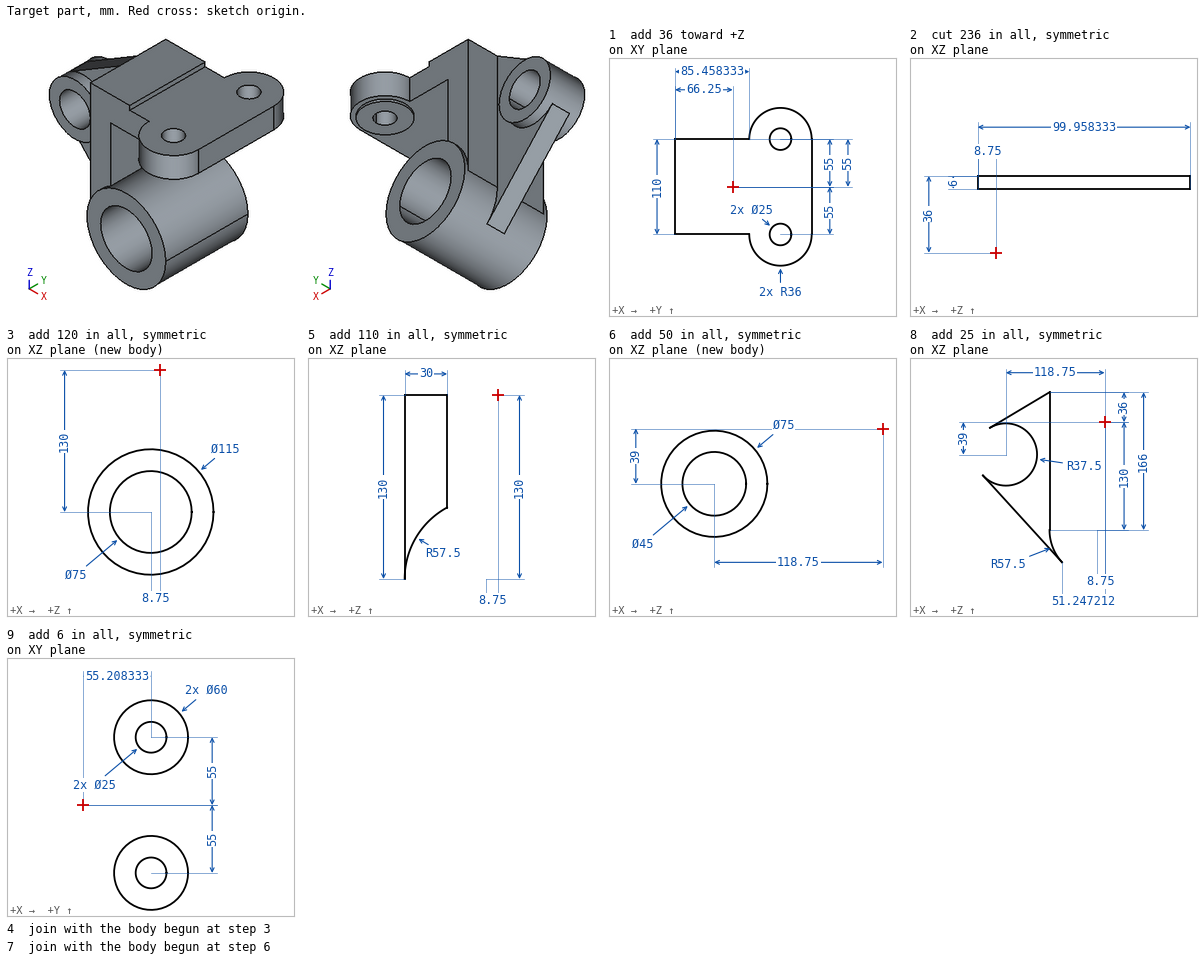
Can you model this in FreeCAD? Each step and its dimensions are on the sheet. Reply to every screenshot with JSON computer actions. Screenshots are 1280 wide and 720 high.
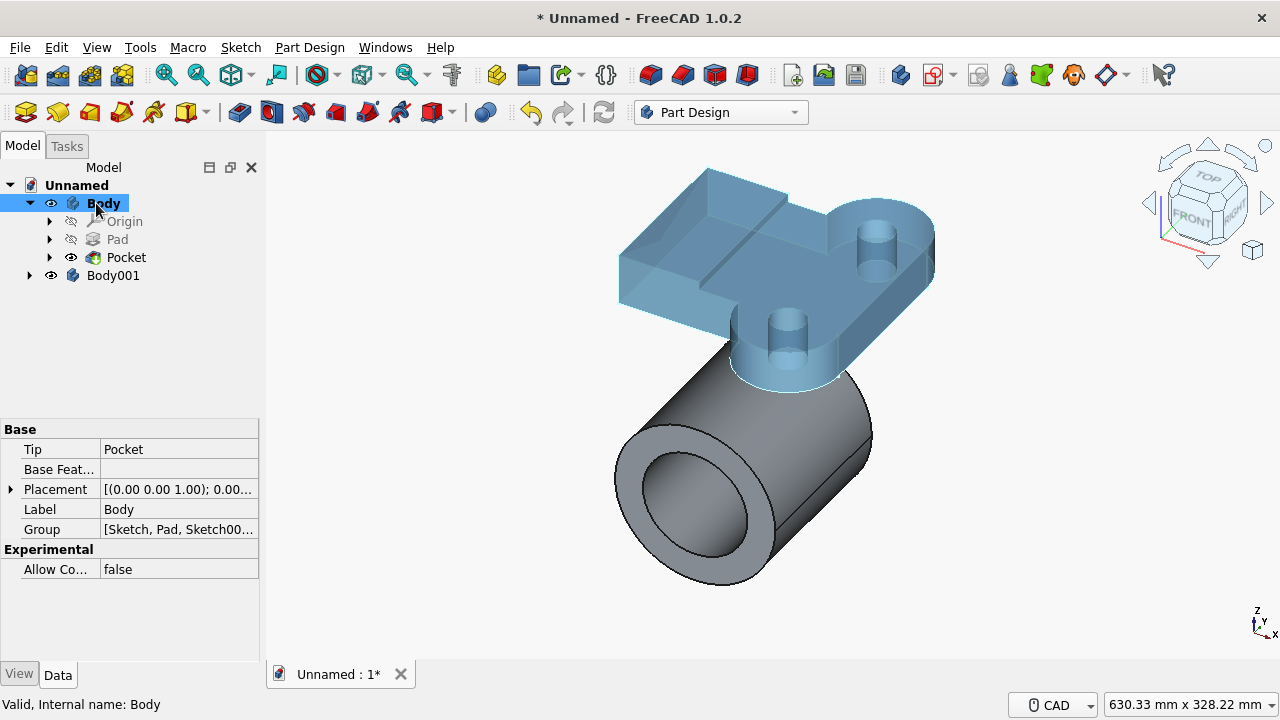
{"action": "left_click", "coordinate": [96, 203]}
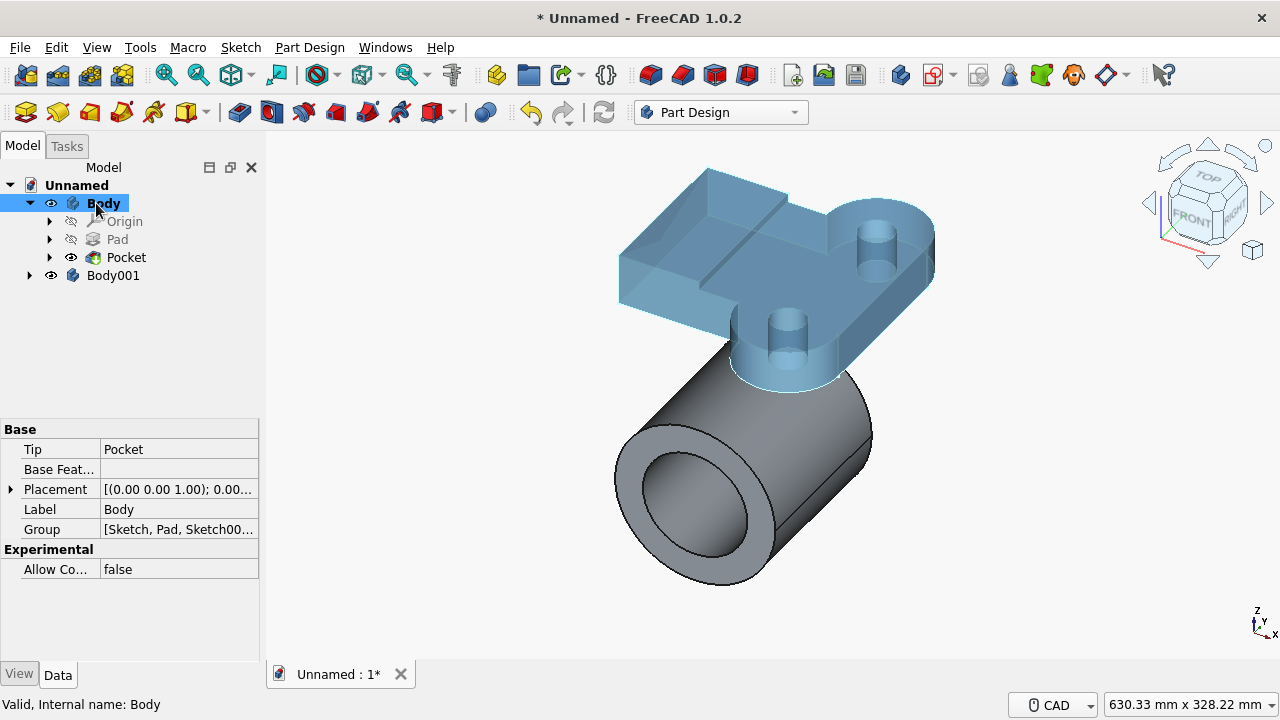
{"action": "left_click", "coordinate": [146, 569]}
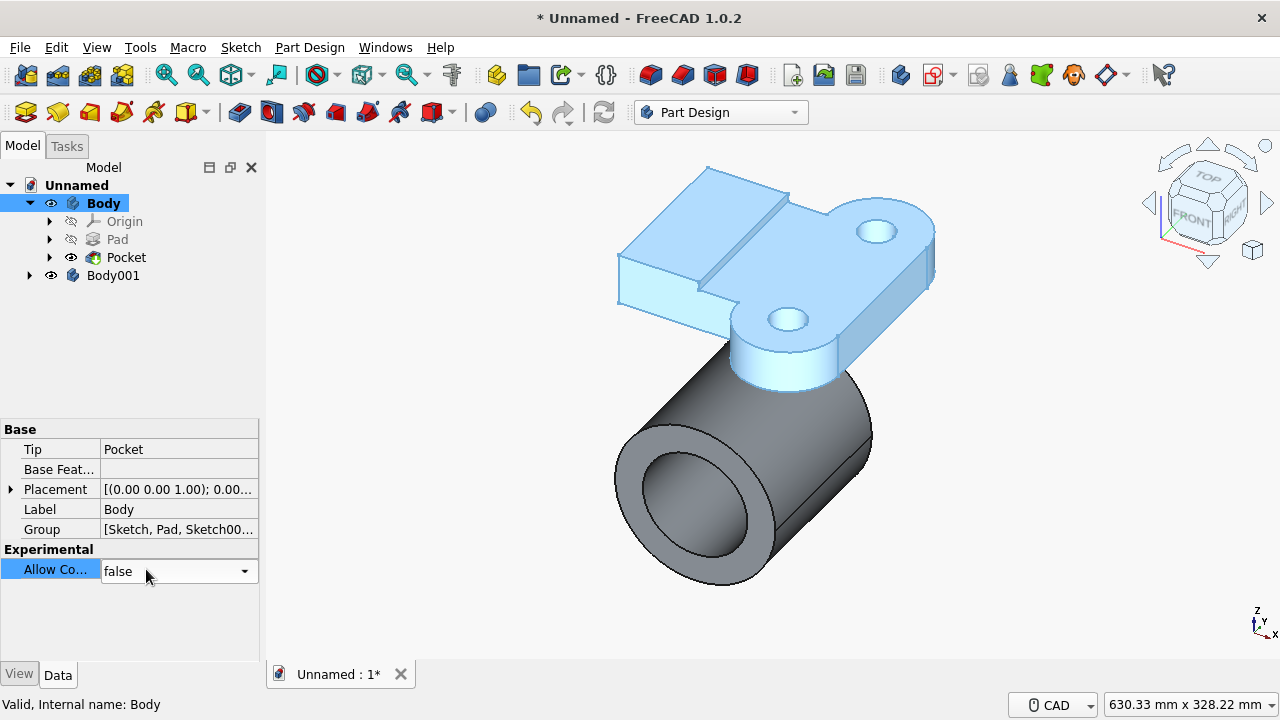
{"action": "left_click", "coordinate": [146, 569]}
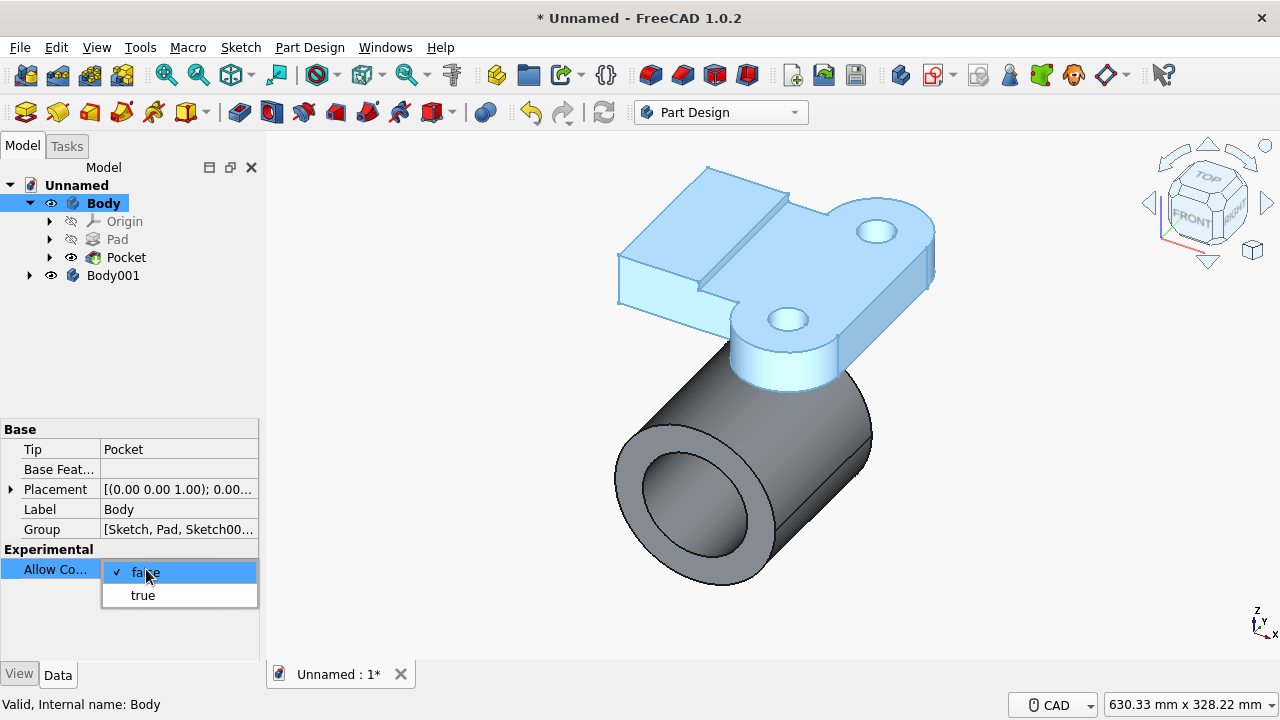
{"action": "left_click", "coordinate": [179, 596]}
{"action": "key", "text": "Return"}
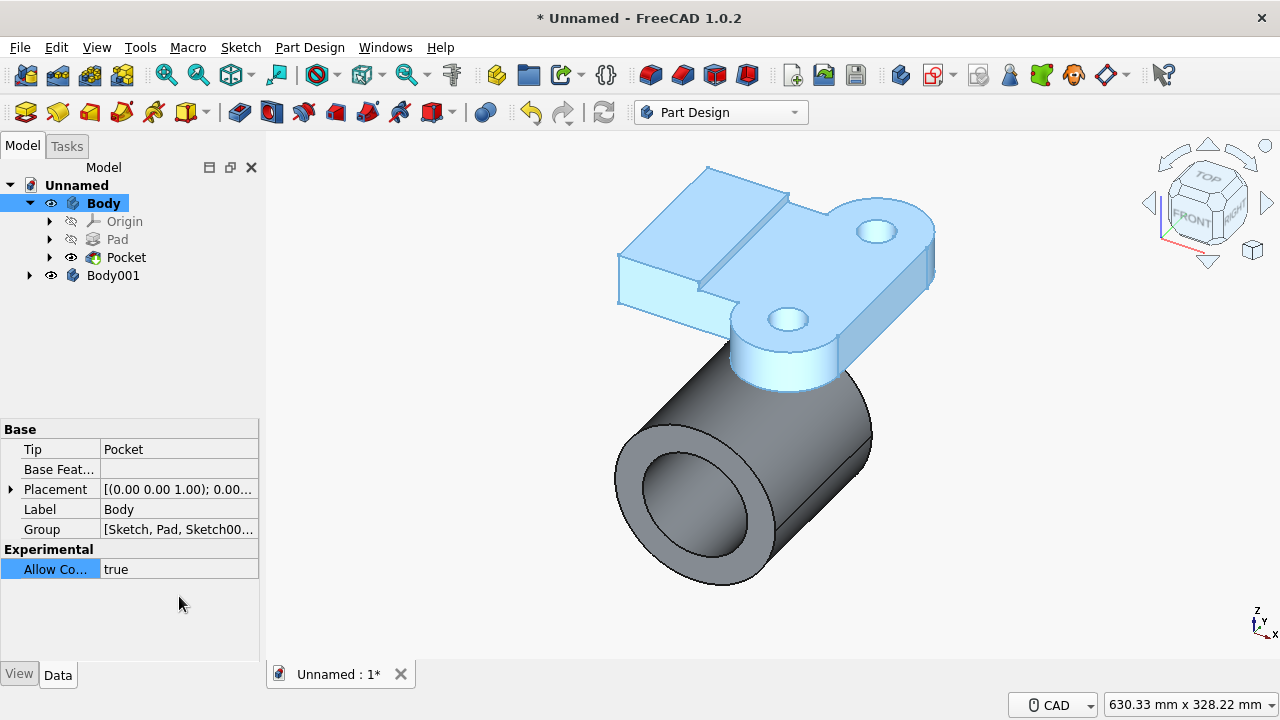
{"action": "left_click", "coordinate": [96, 275]}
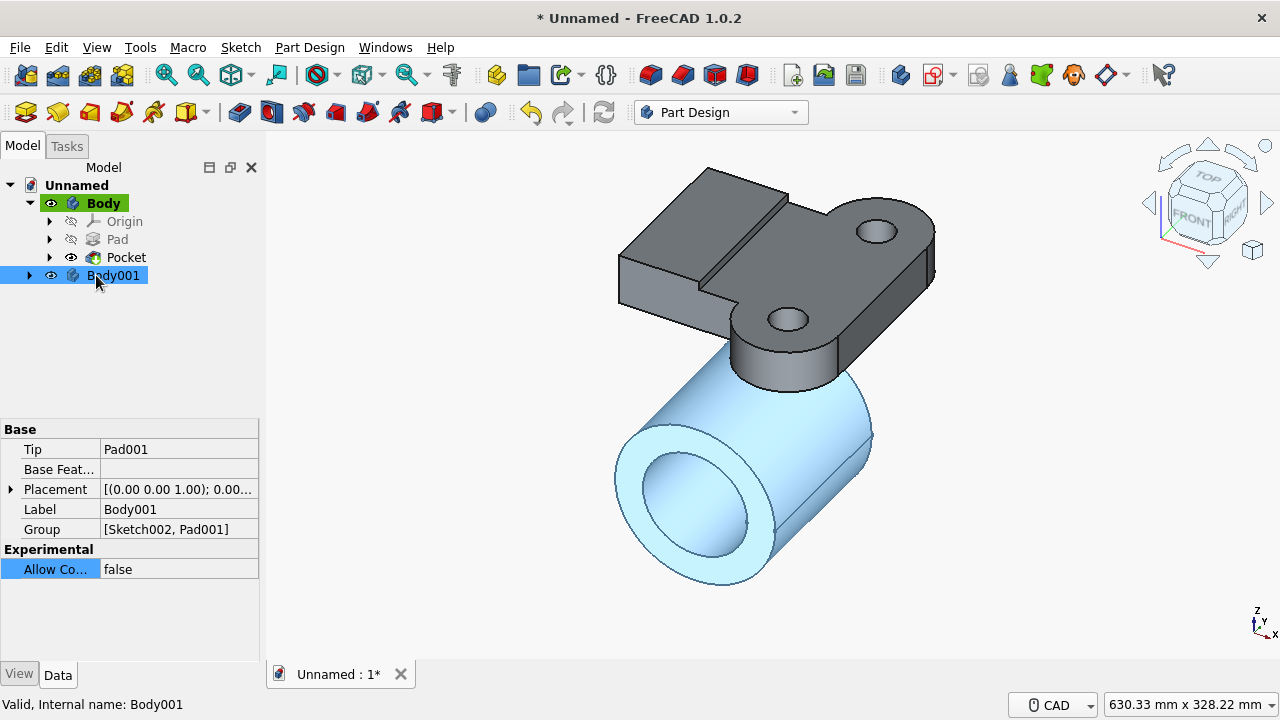
{"action": "left_click", "coordinate": [486, 112]}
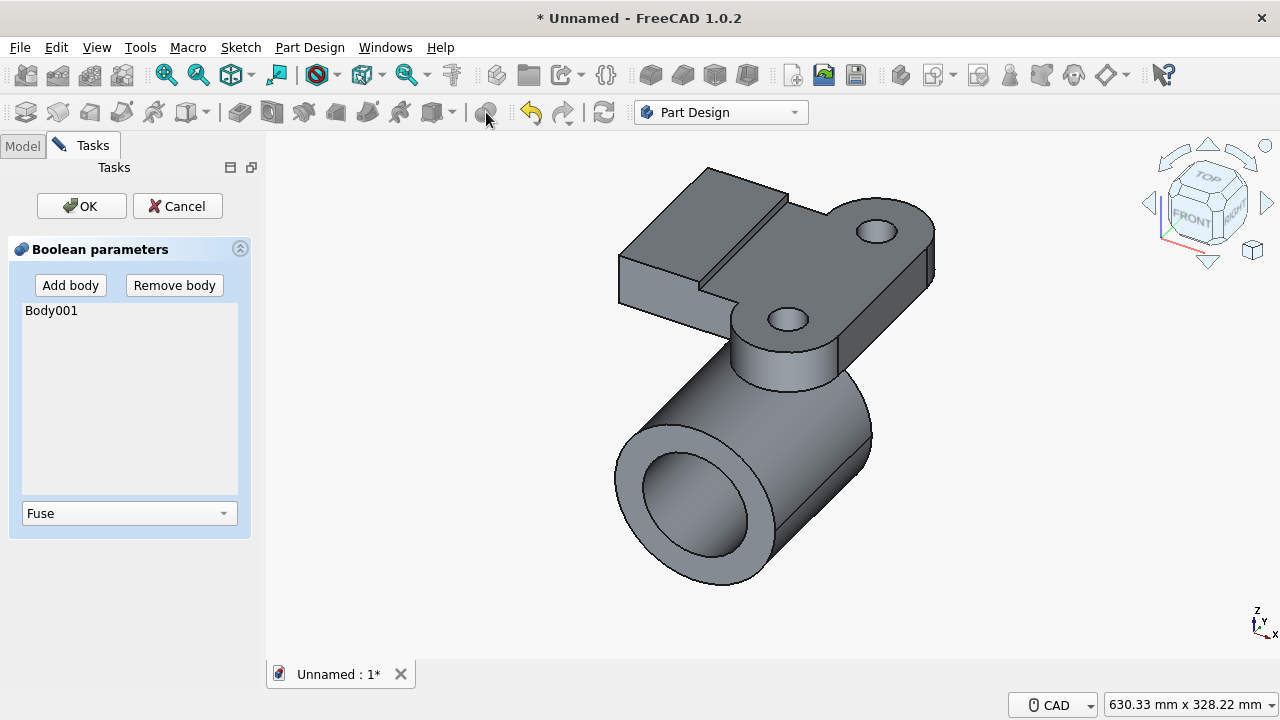
{"action": "left_click", "coordinate": [82, 206]}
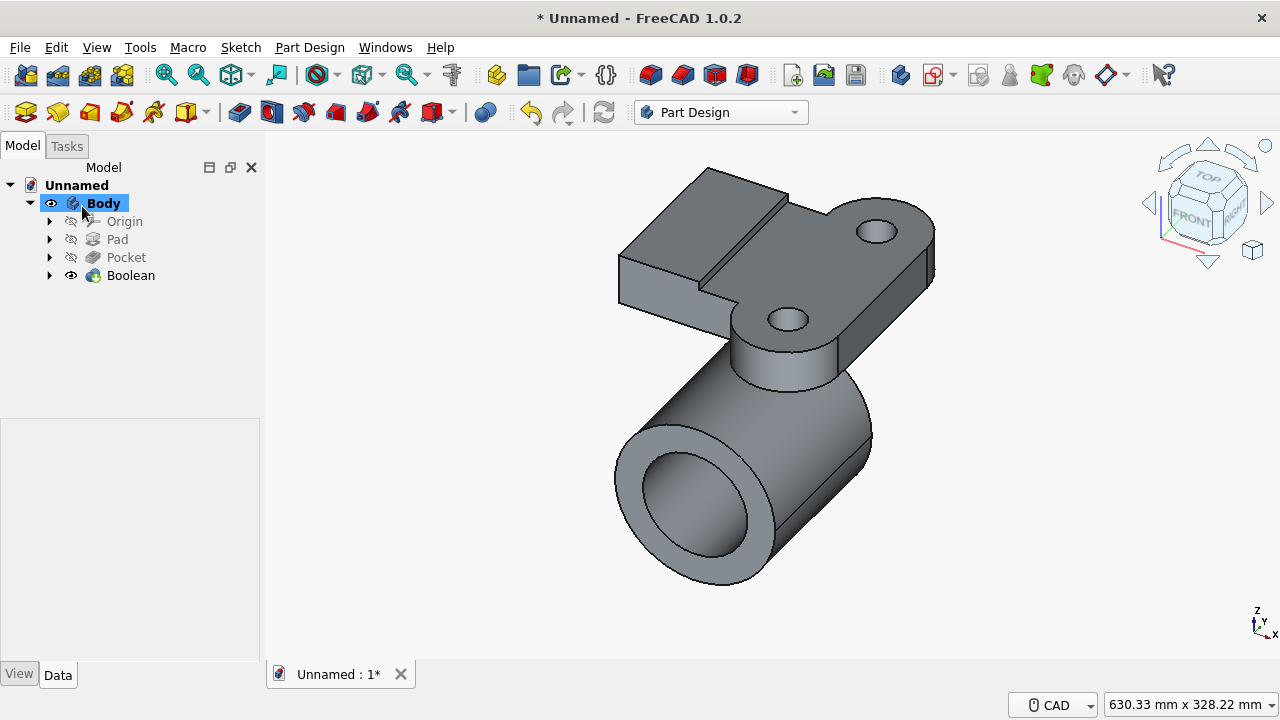
{"action": "left_click", "coordinate": [934, 76]}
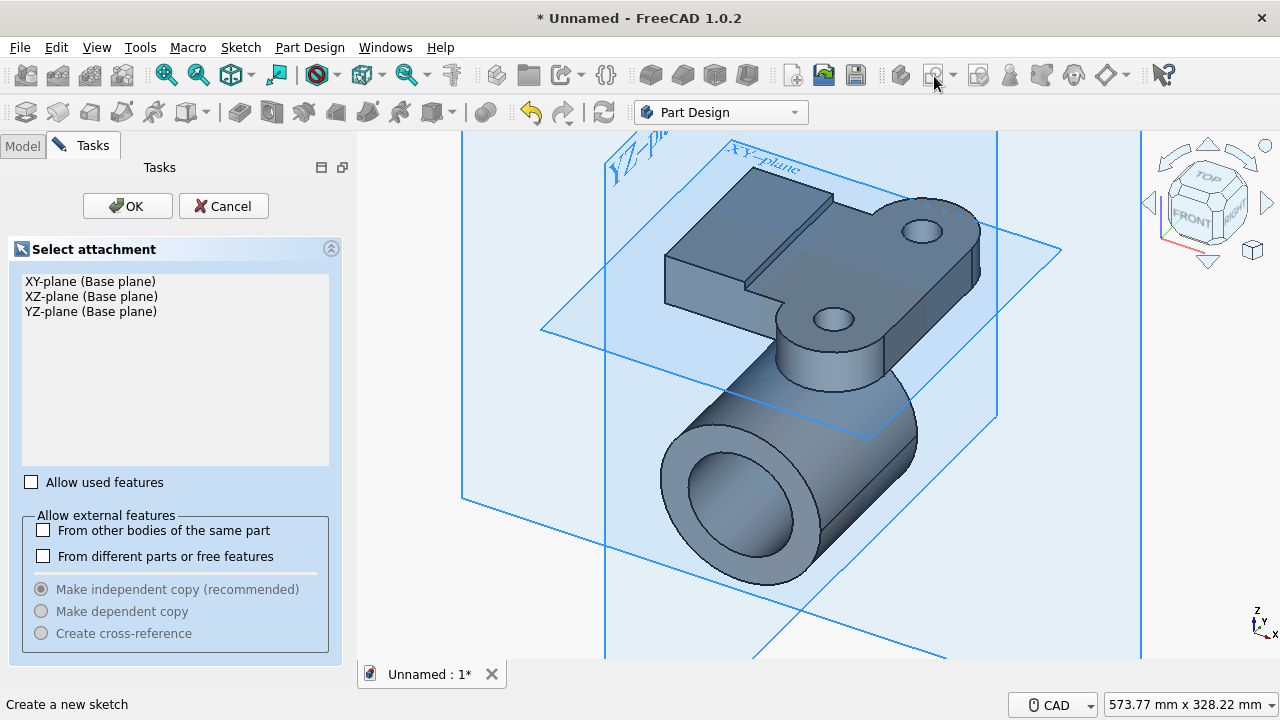
{"action": "left_click", "coordinate": [82, 296]}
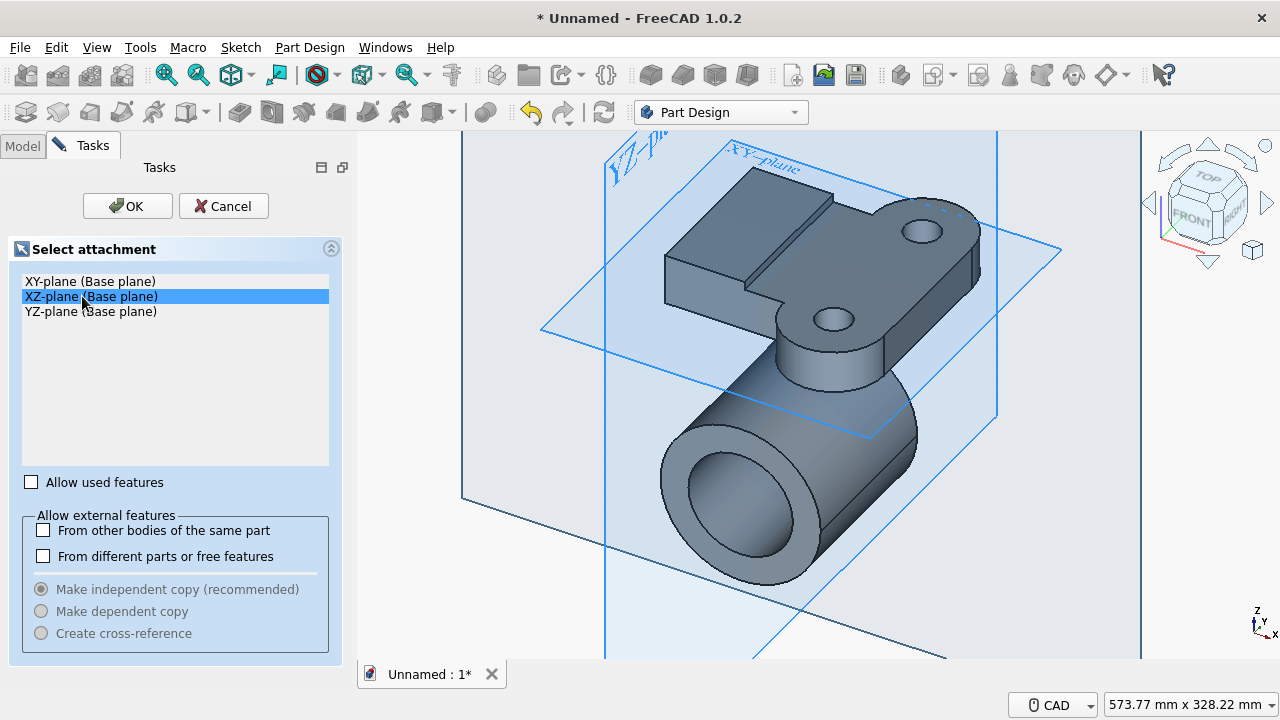
{"action": "left_click", "coordinate": [128, 206]}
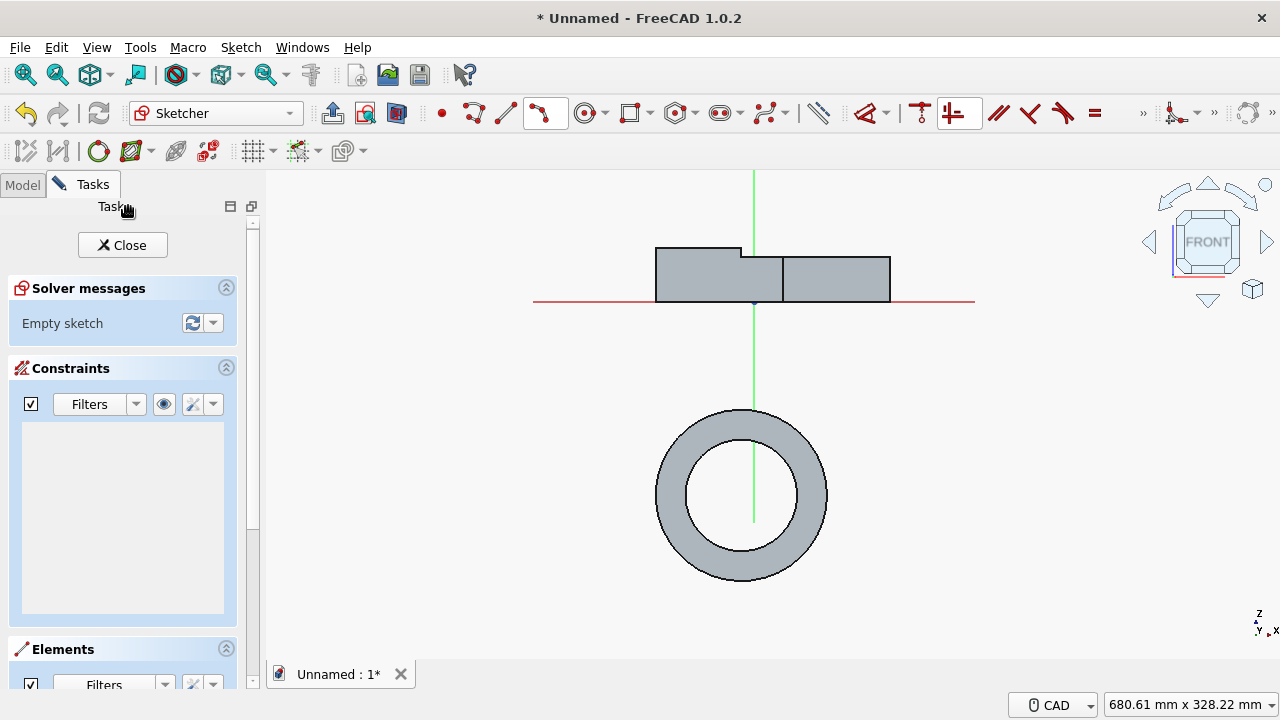
{"action": "left_click", "coordinate": [398, 114]}